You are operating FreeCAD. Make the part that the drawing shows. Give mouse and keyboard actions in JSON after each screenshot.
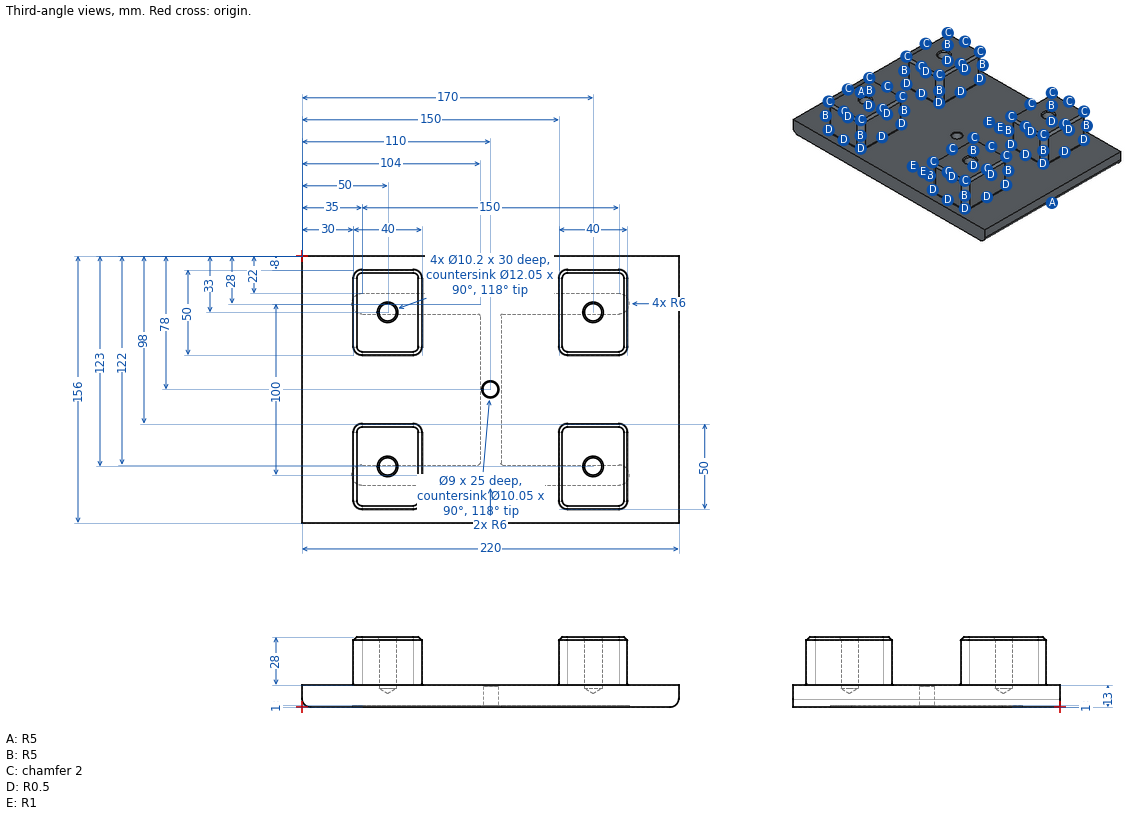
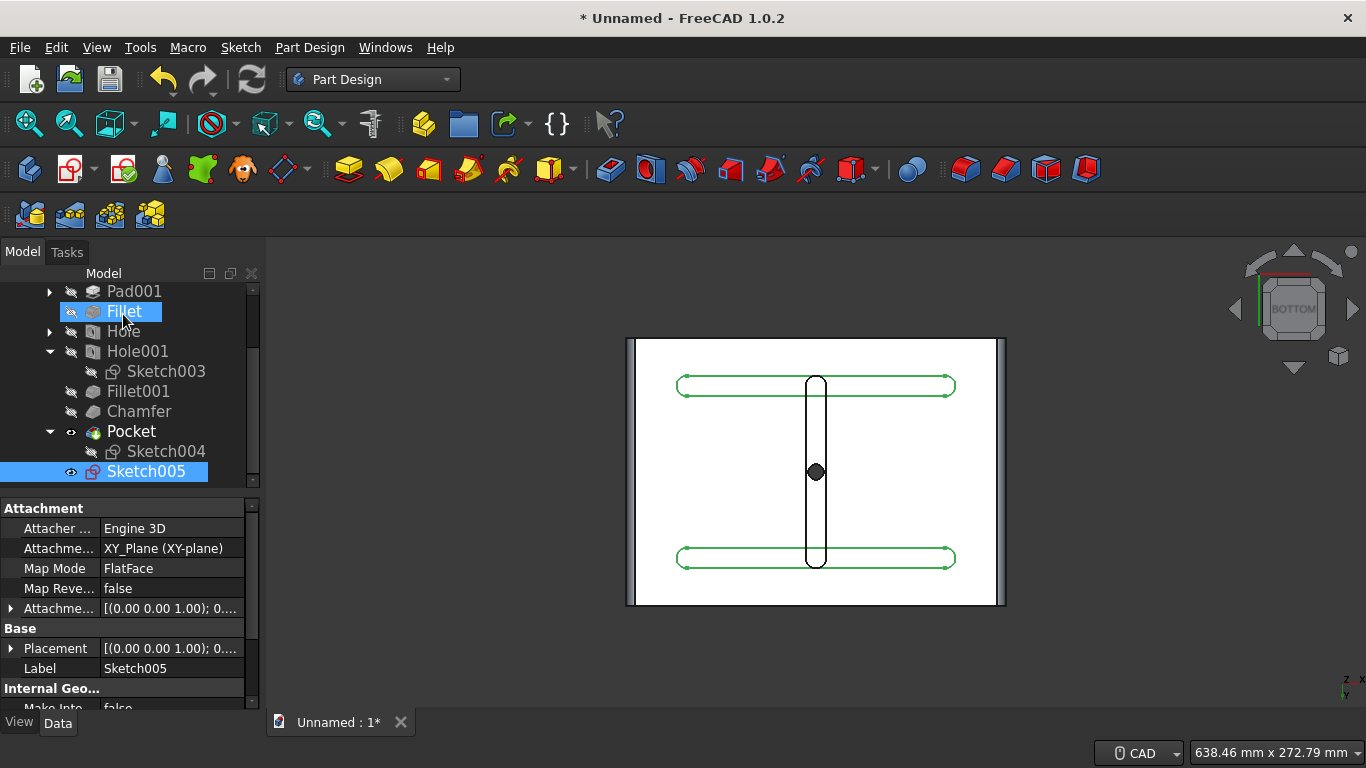
{"action": "left_click", "coordinate": [612, 170]}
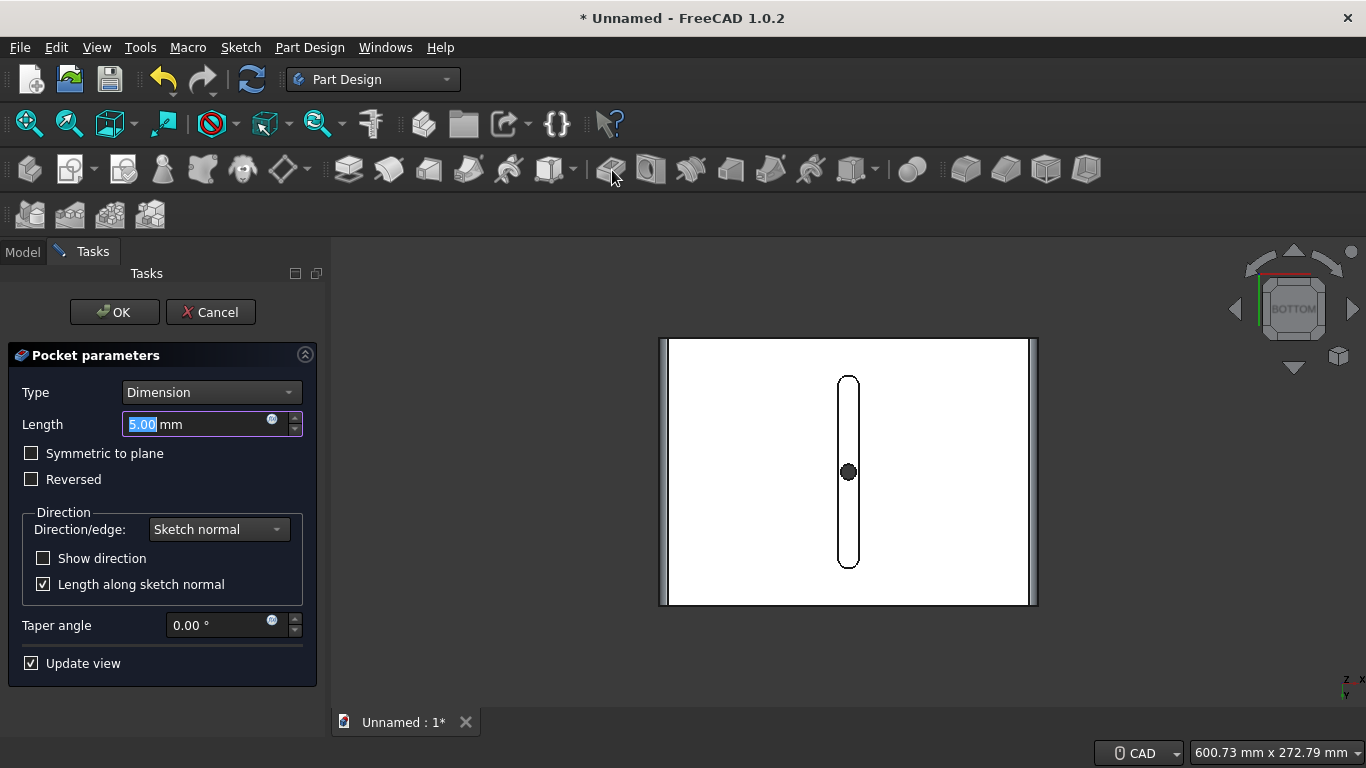
{"action": "type", "text": "1"}
{"action": "key", "text": "Tab"}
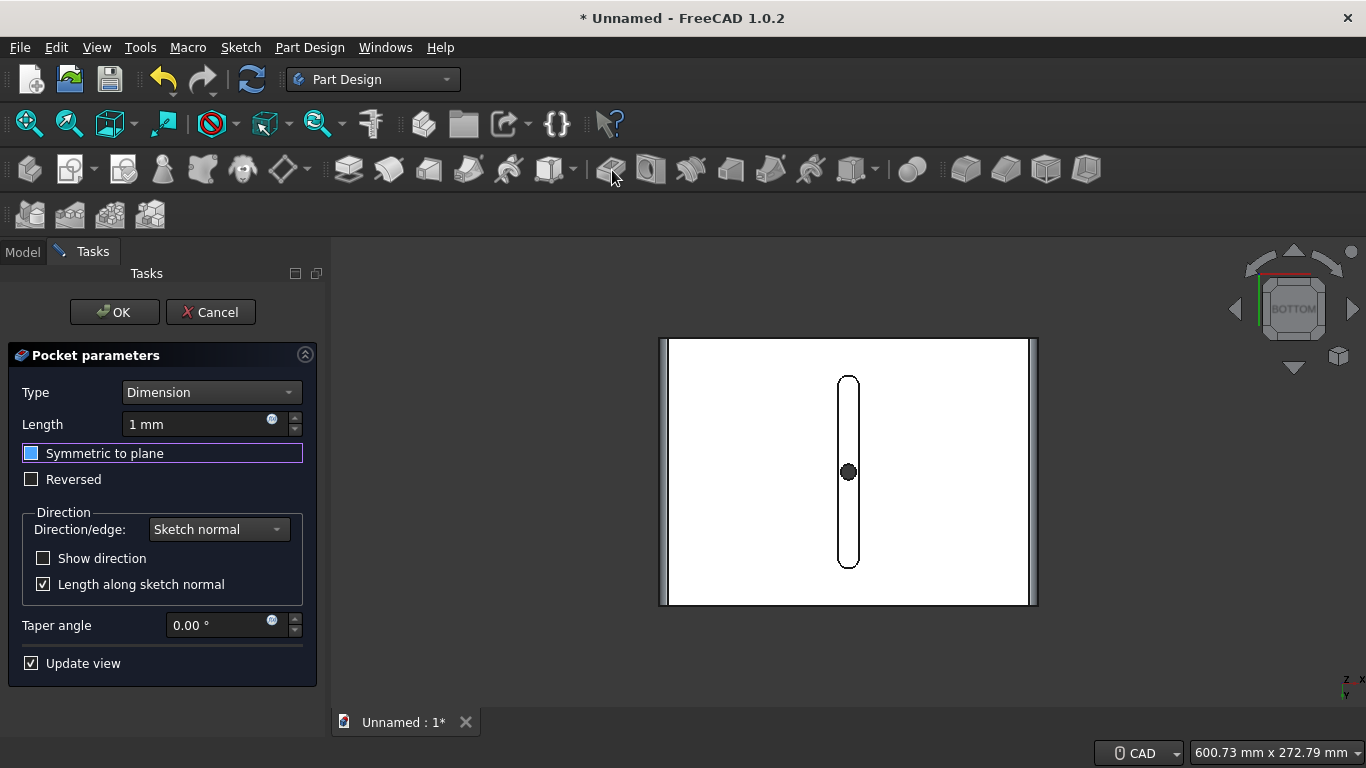
{"action": "left_click", "coordinate": [30, 479]}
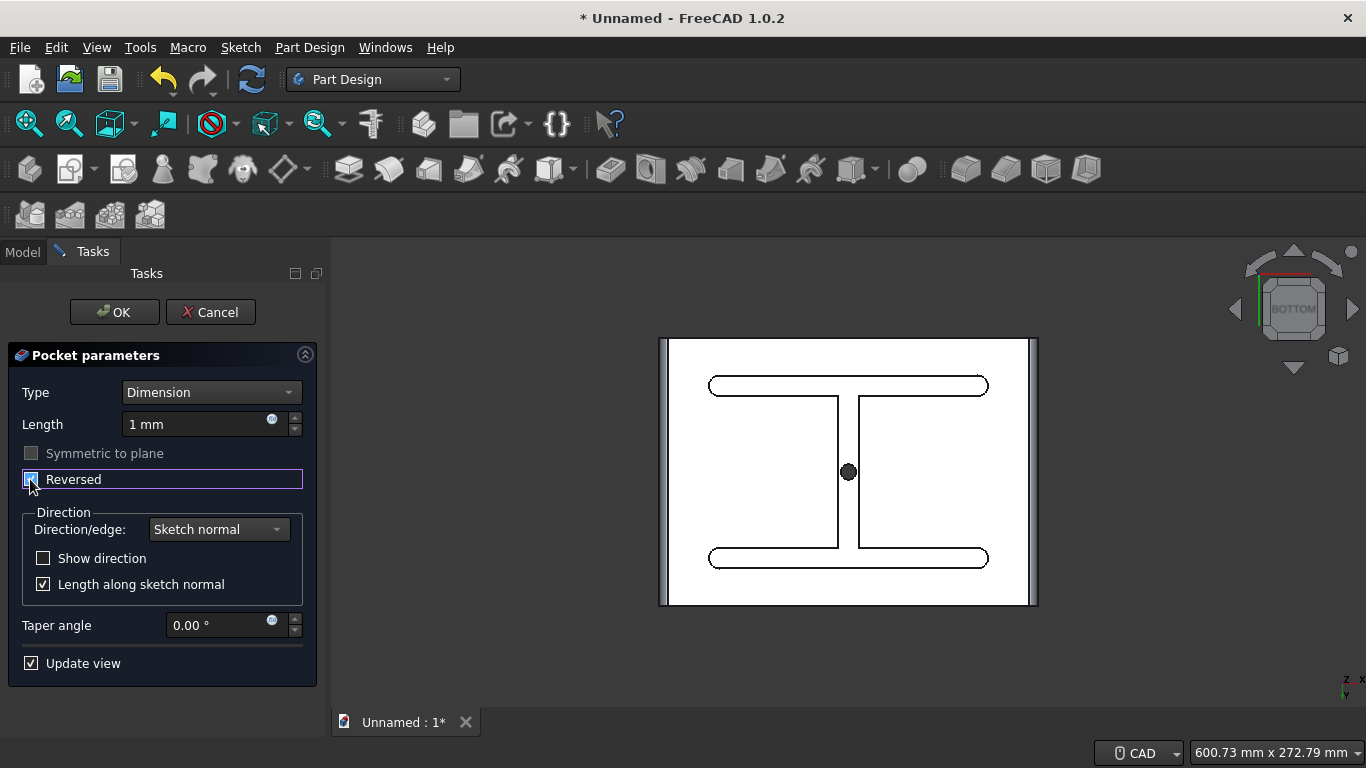
{"action": "left_click", "coordinate": [115, 312]}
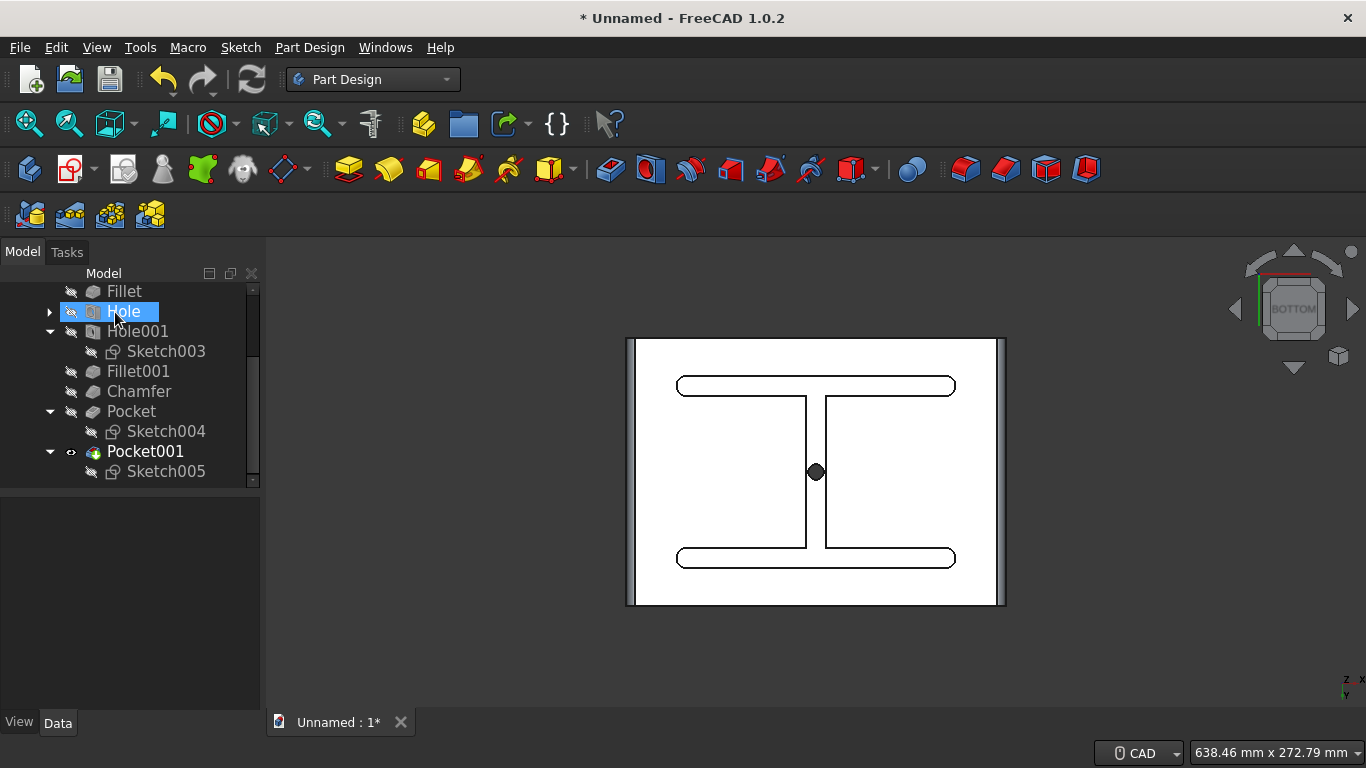
{"action": "key", "text": "0"}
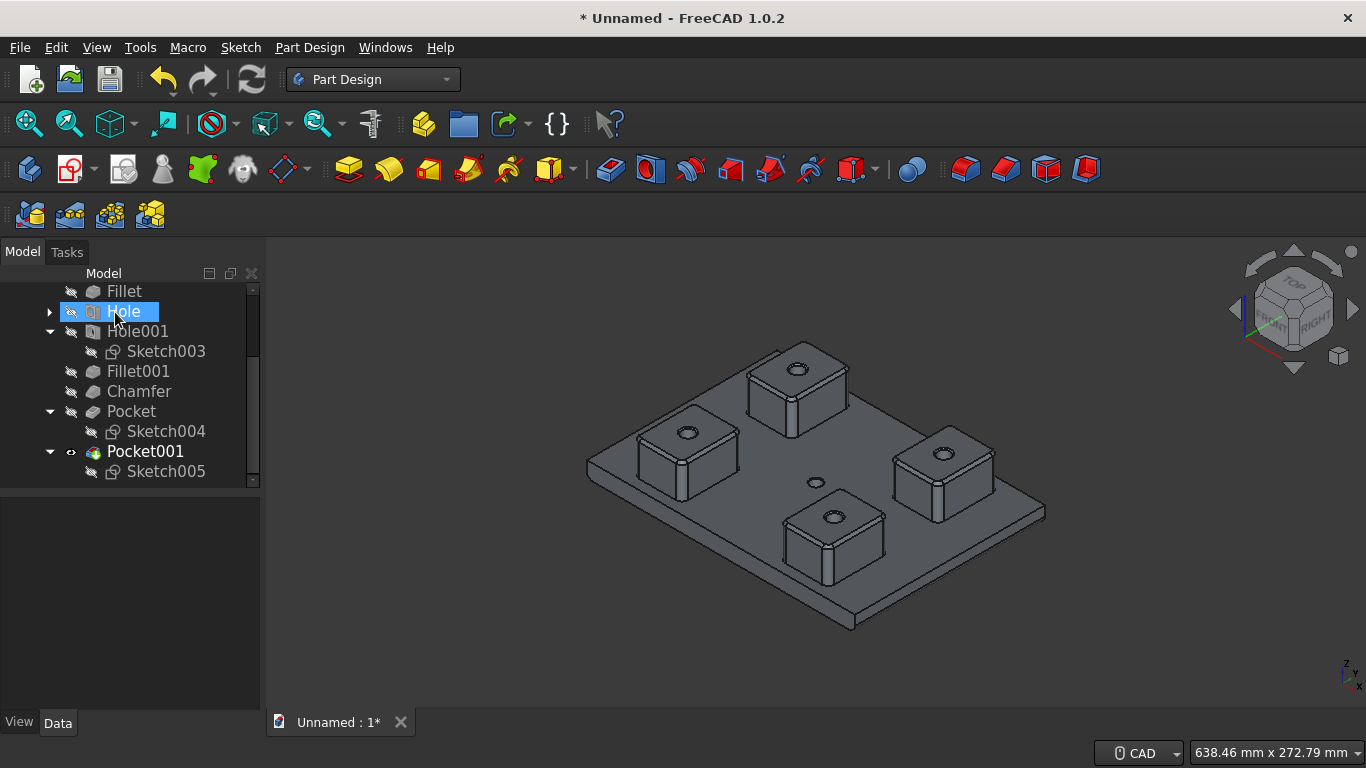
{"action": "left_click", "coordinate": [676, 499]}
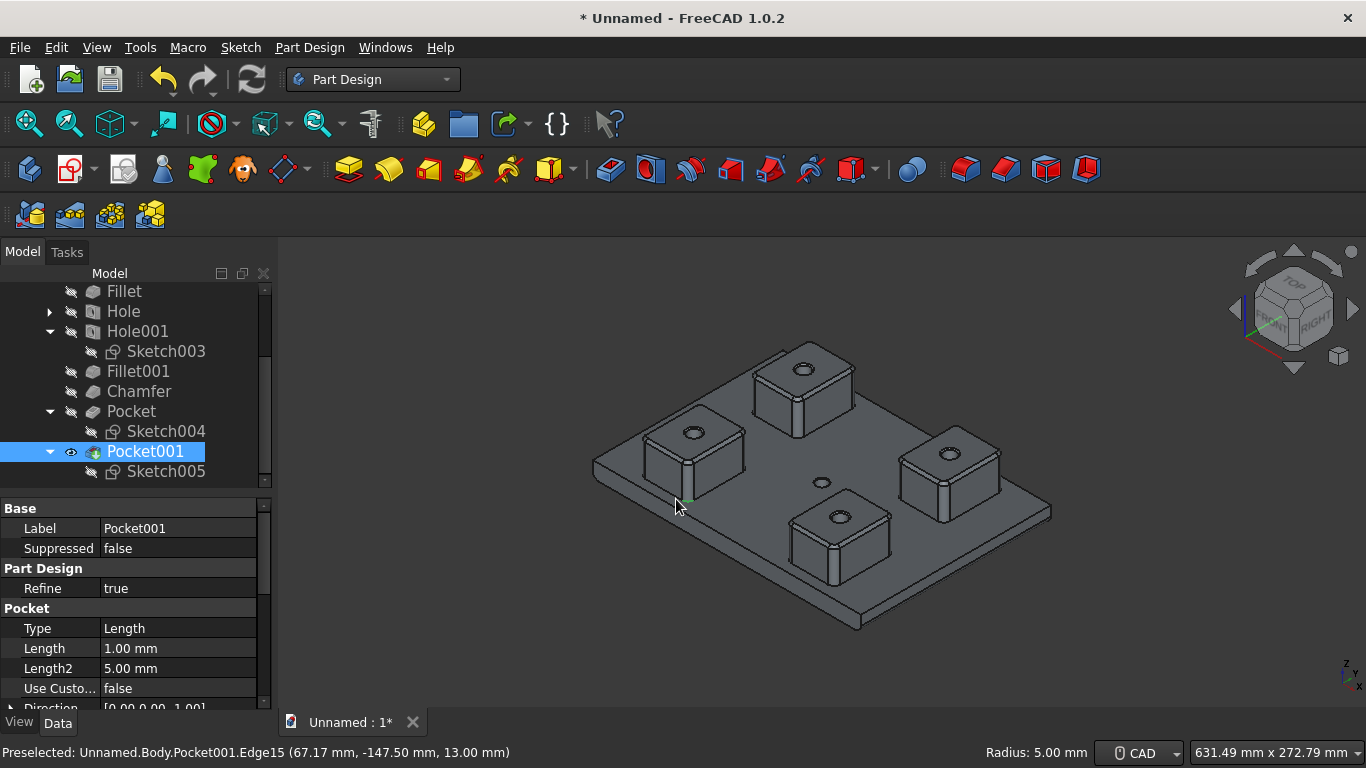
{"action": "left_click", "coordinate": [792, 436], "text": "ctrl"}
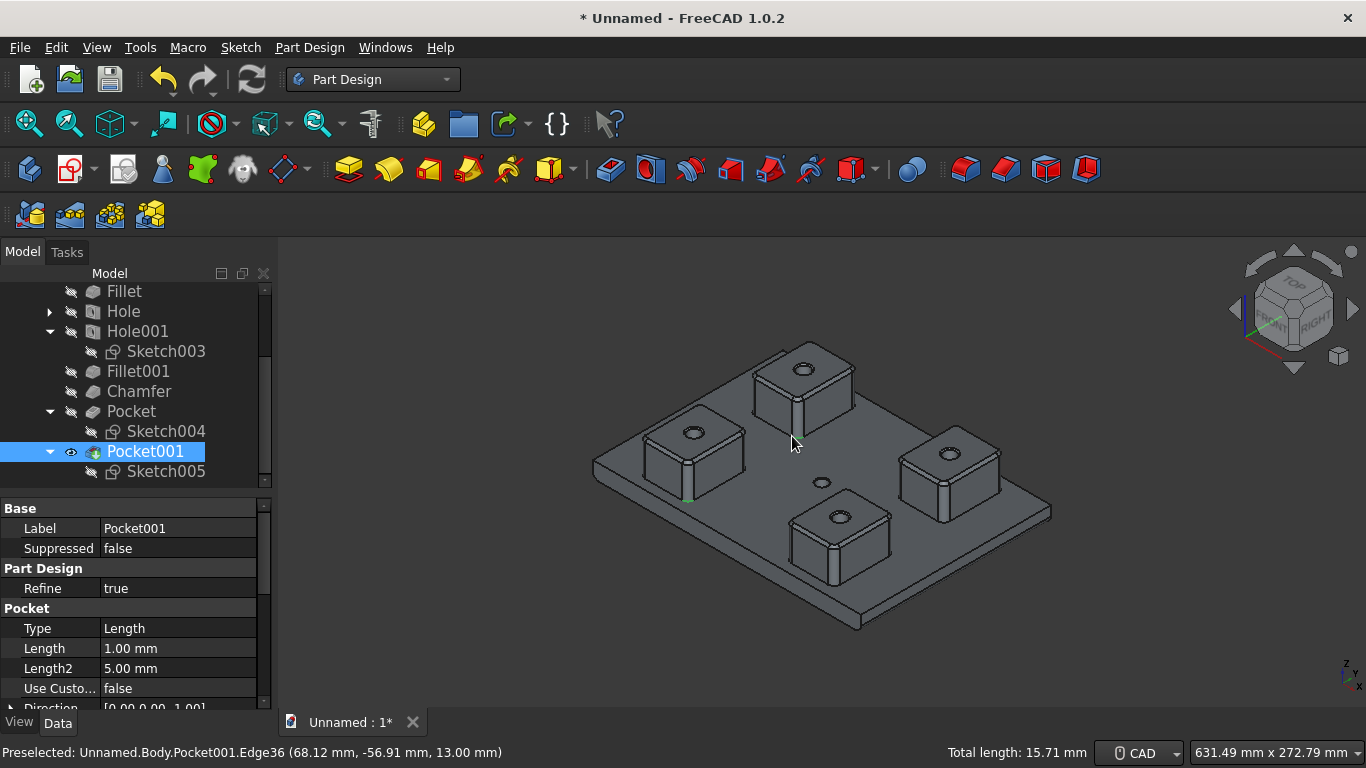
{"action": "key", "text": "2"}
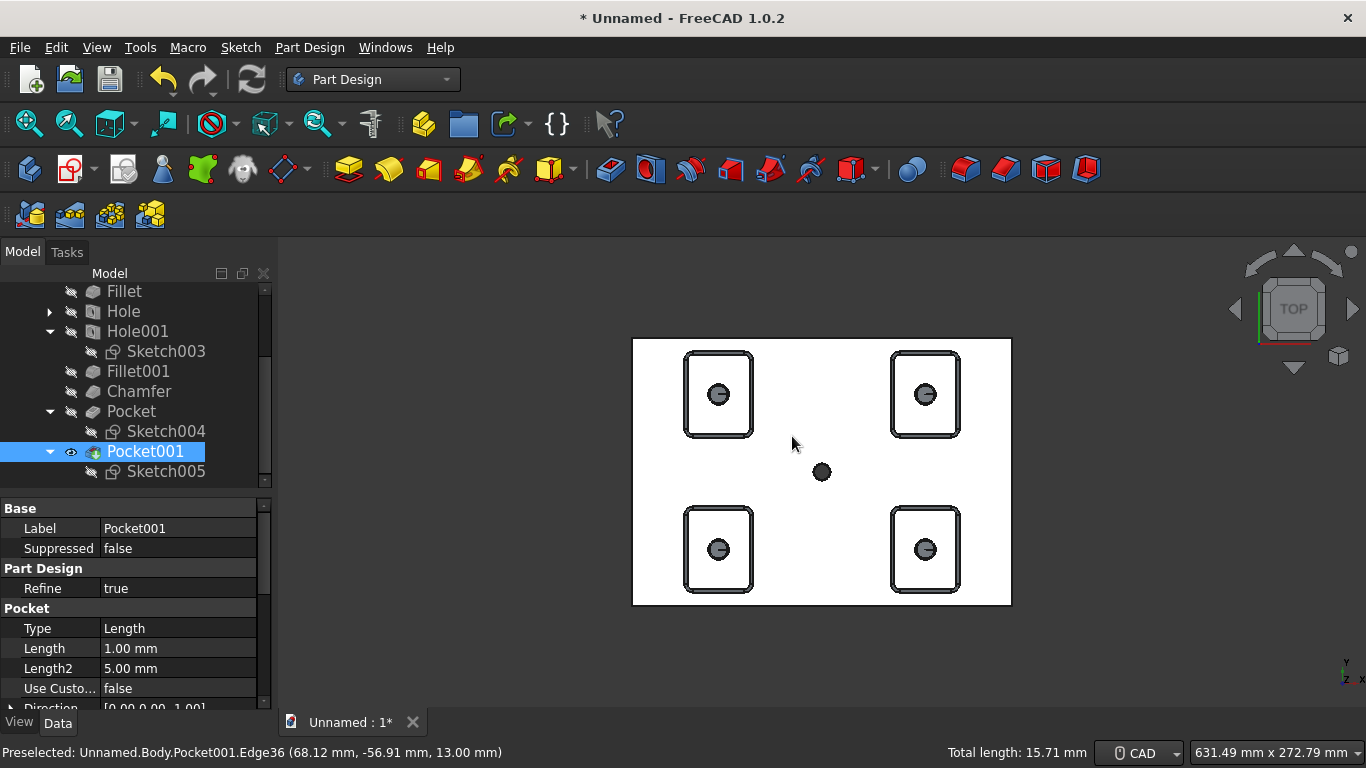
{"action": "key", "text": "1"}